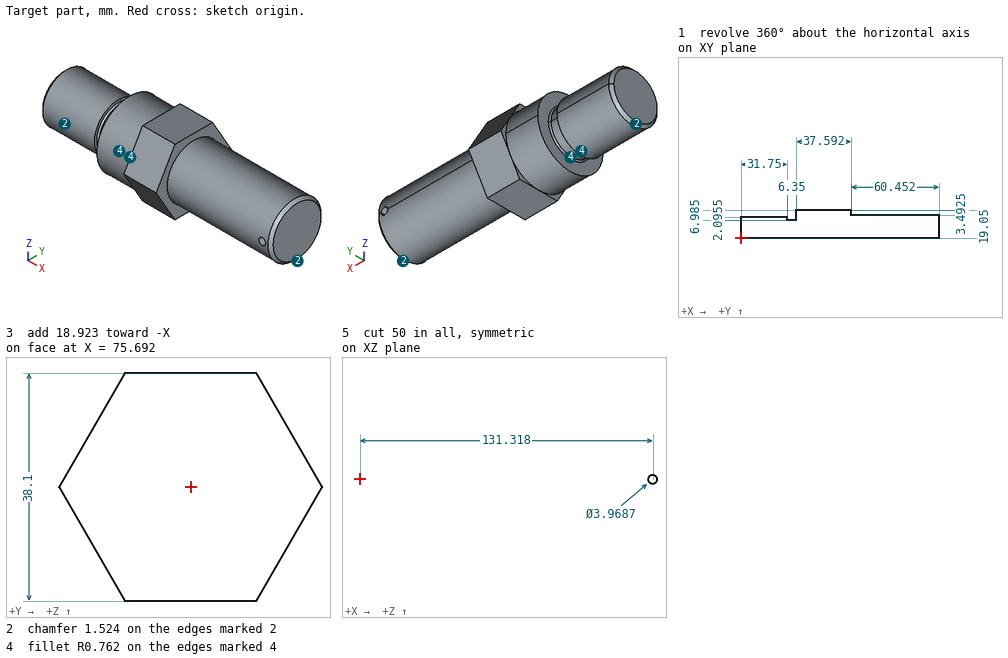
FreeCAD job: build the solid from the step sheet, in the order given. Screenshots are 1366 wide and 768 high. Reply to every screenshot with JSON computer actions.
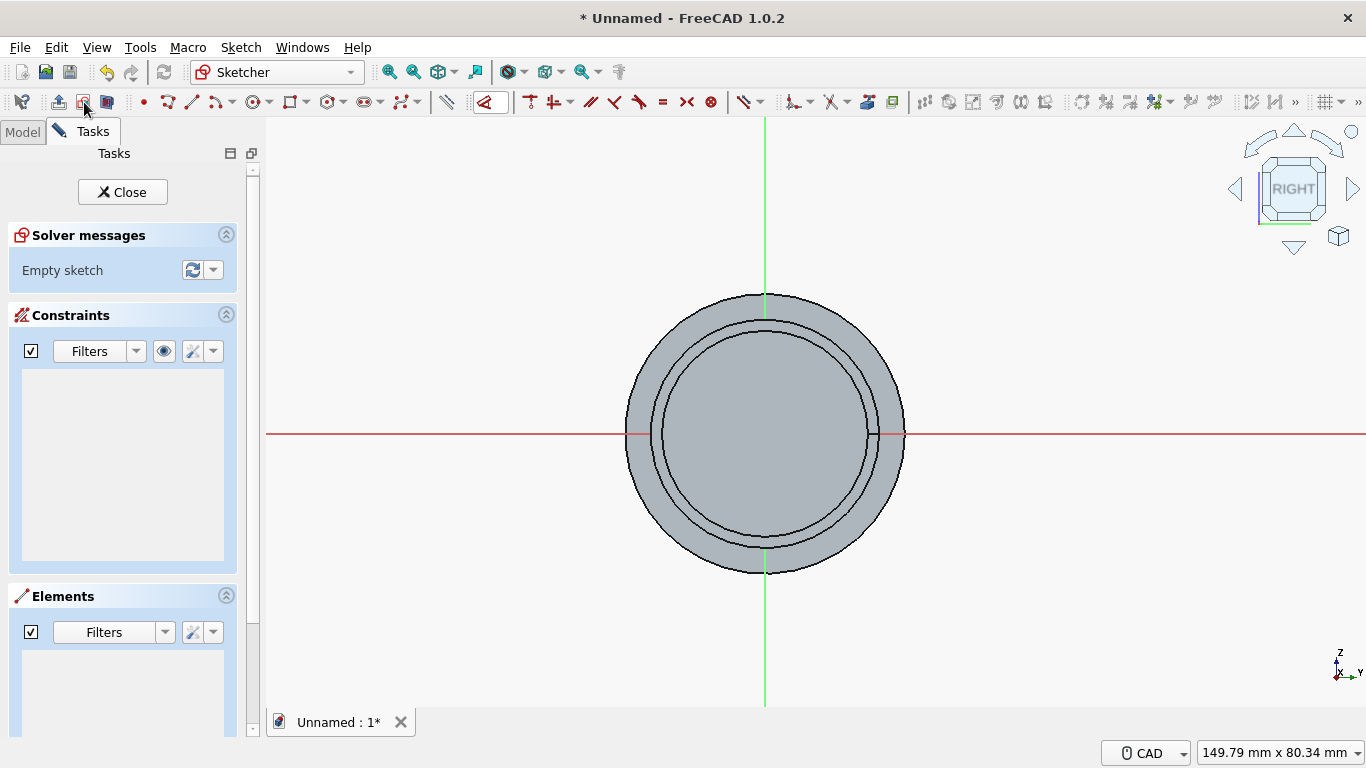
{"action": "key", "text": "q s"}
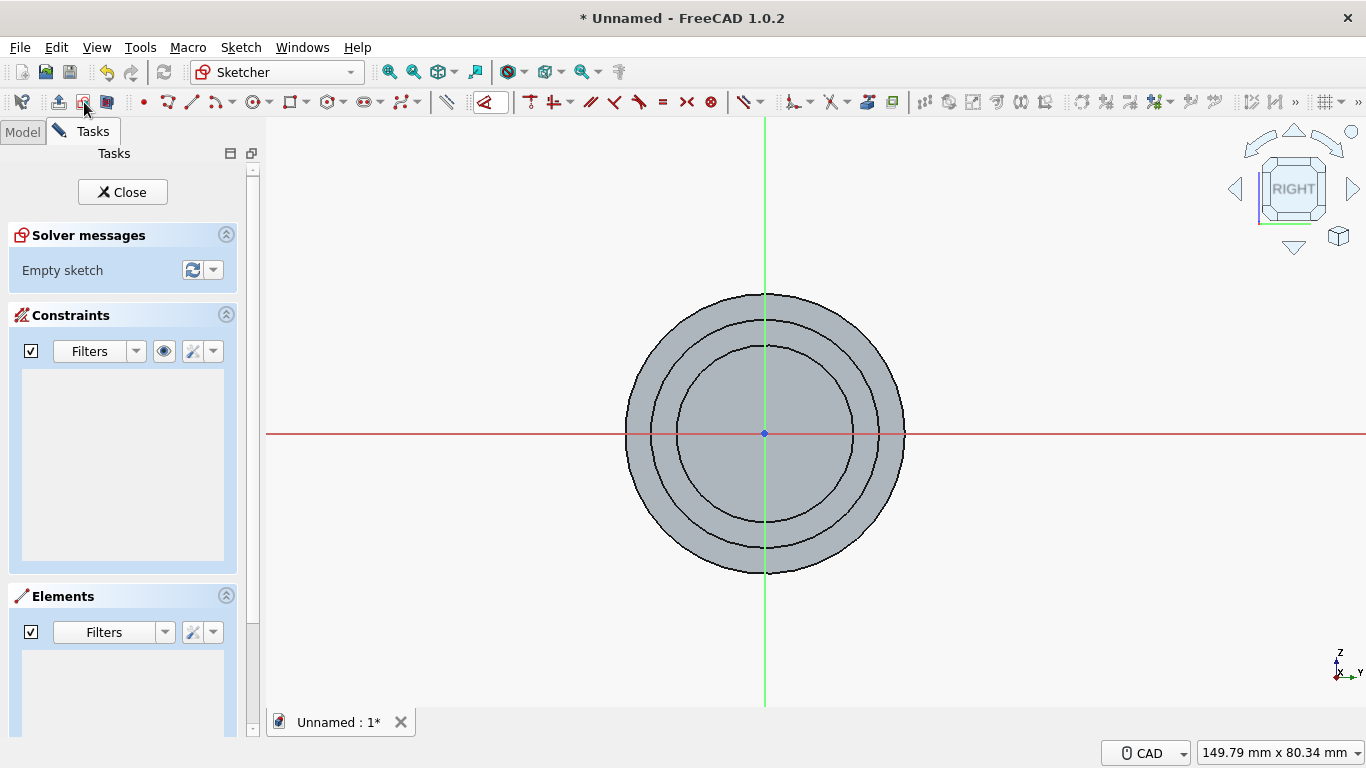
{"action": "key", "text": "g p 6"}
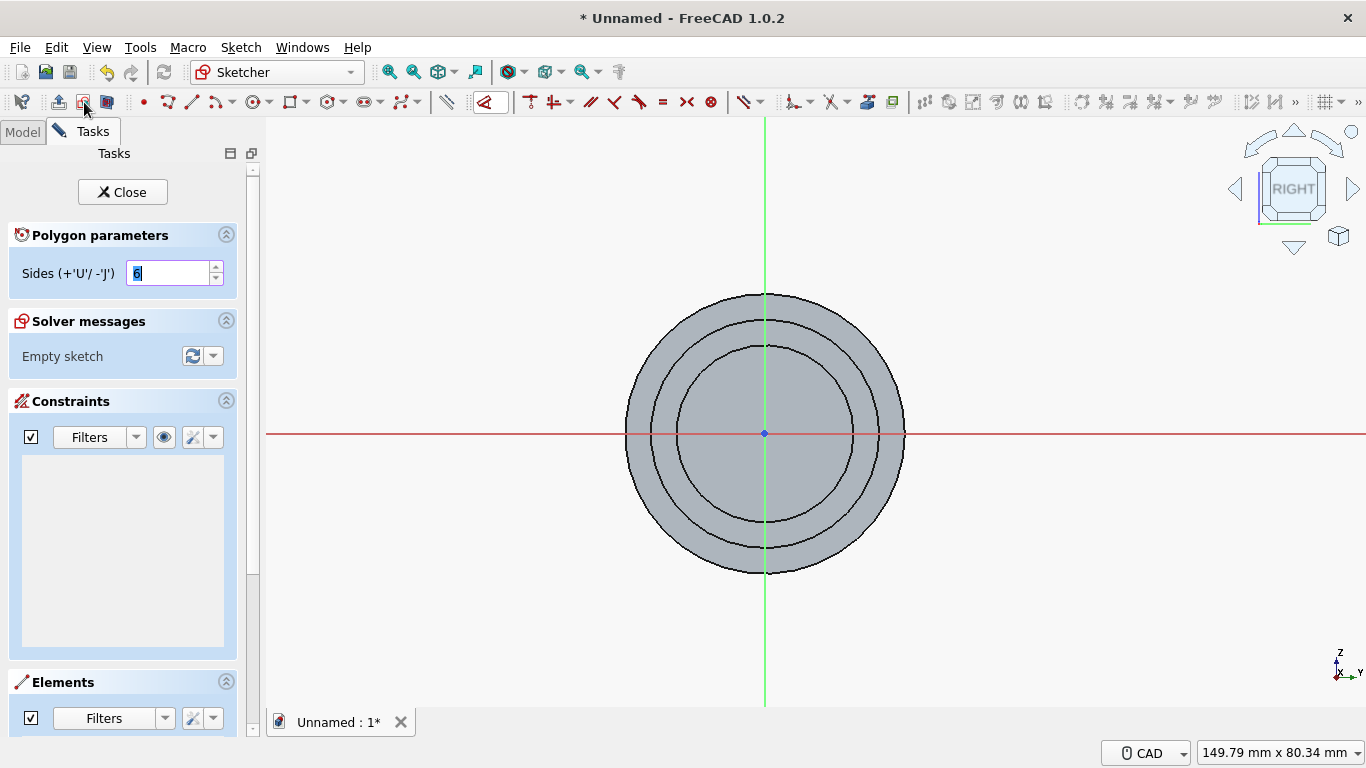
{"action": "left_click", "coordinate": [765, 434]}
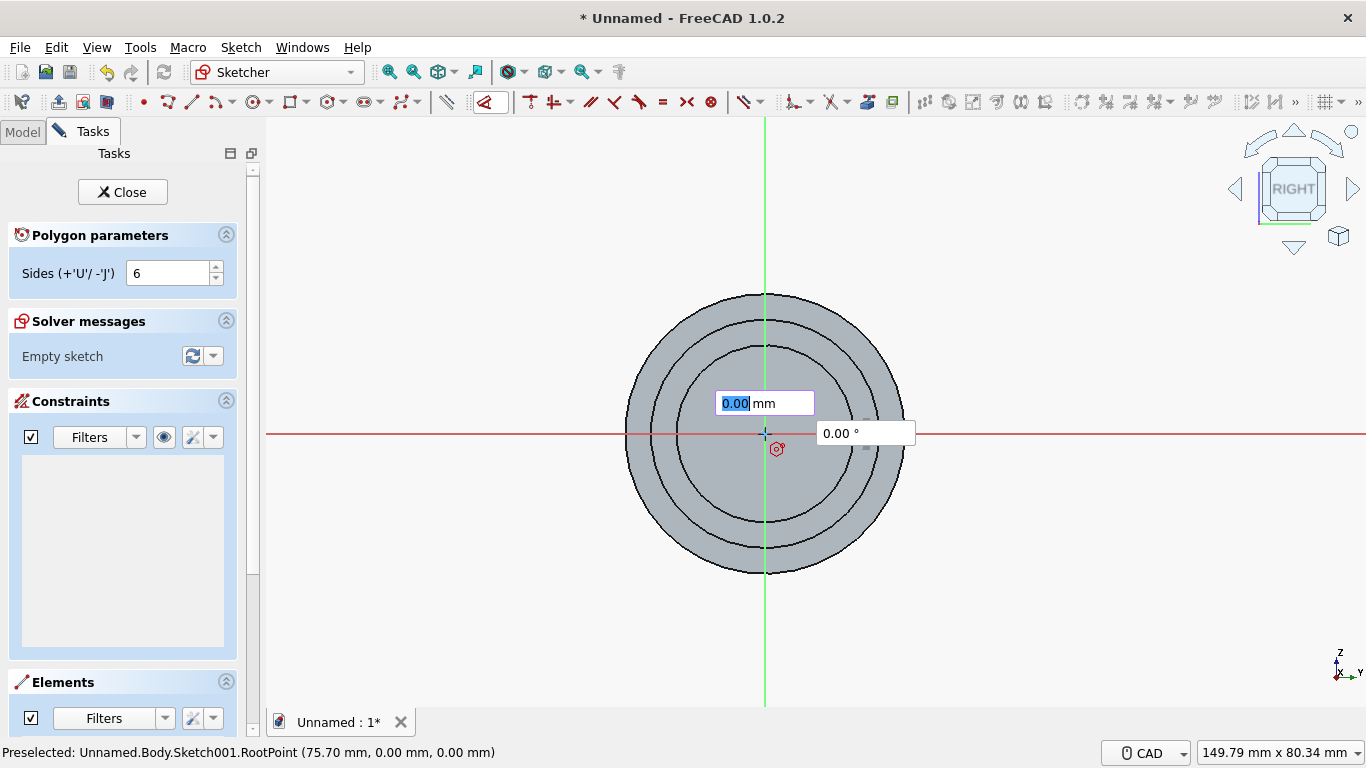
{"action": "left_click", "coordinate": [927, 434]}
{"action": "right_click", "coordinate": [927, 434]}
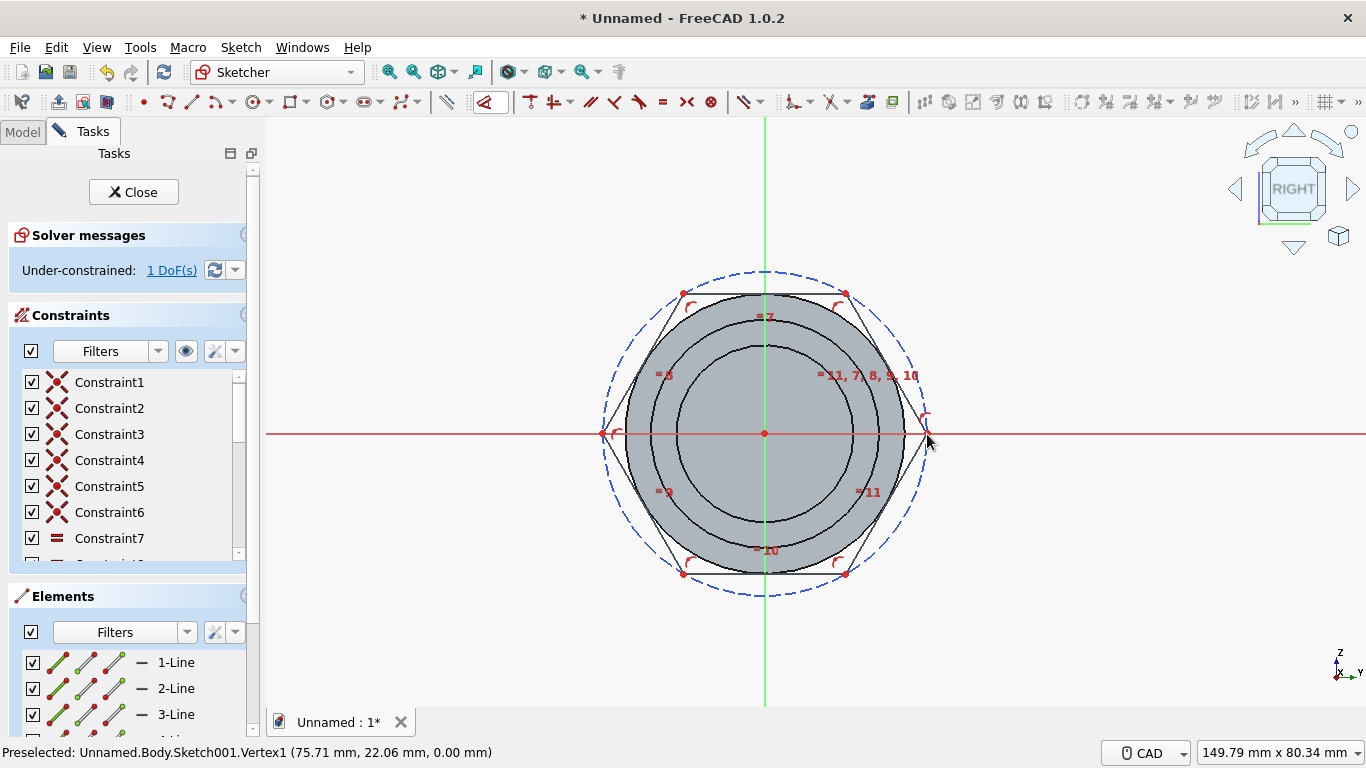
{"action": "left_click", "coordinate": [484, 102]}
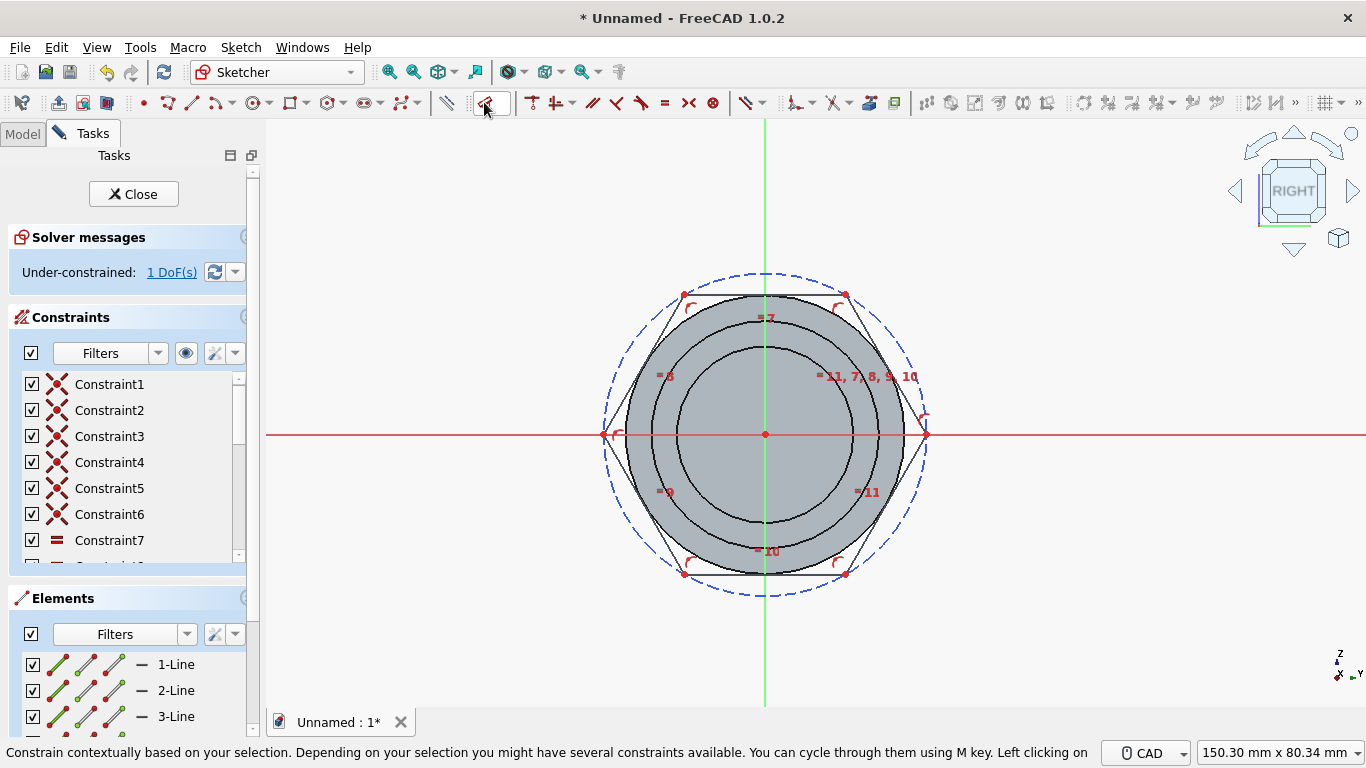
{"action": "left_click", "coordinate": [684, 575]}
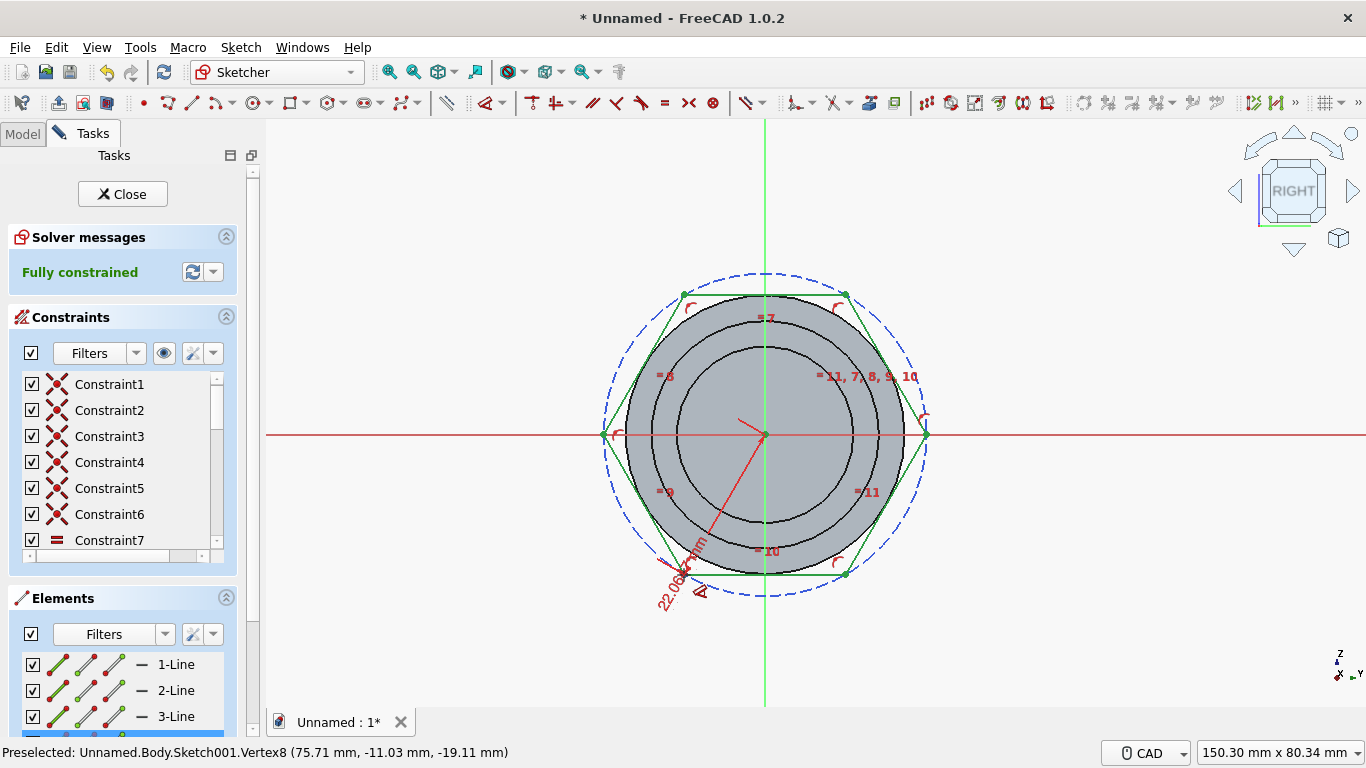
{"action": "left_click", "coordinate": [846, 295]}
{"action": "left_click", "coordinate": [928, 370]}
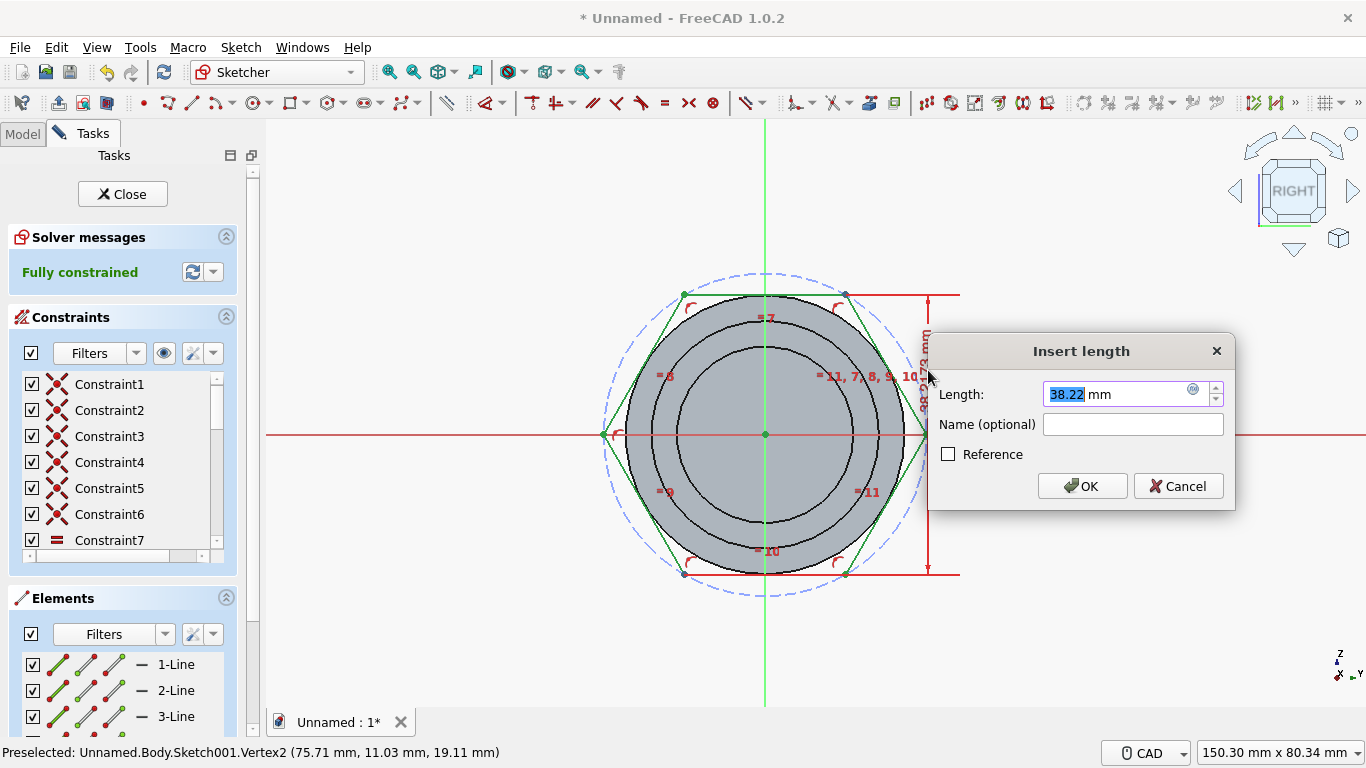
{"action": "type", "text": "38.1"}
{"action": "key", "text": "Return"}
{"action": "key", "text": "Escape"}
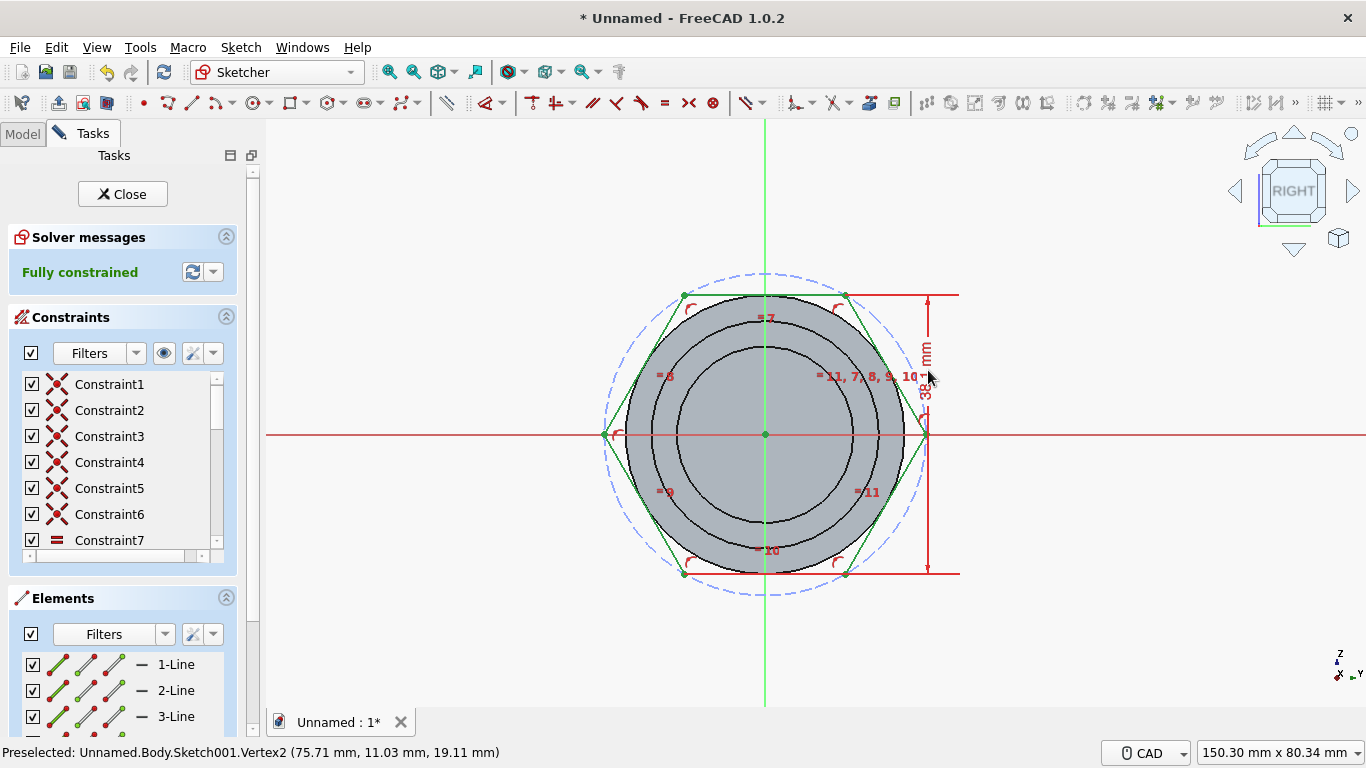
{"action": "left_click", "coordinate": [123, 194]}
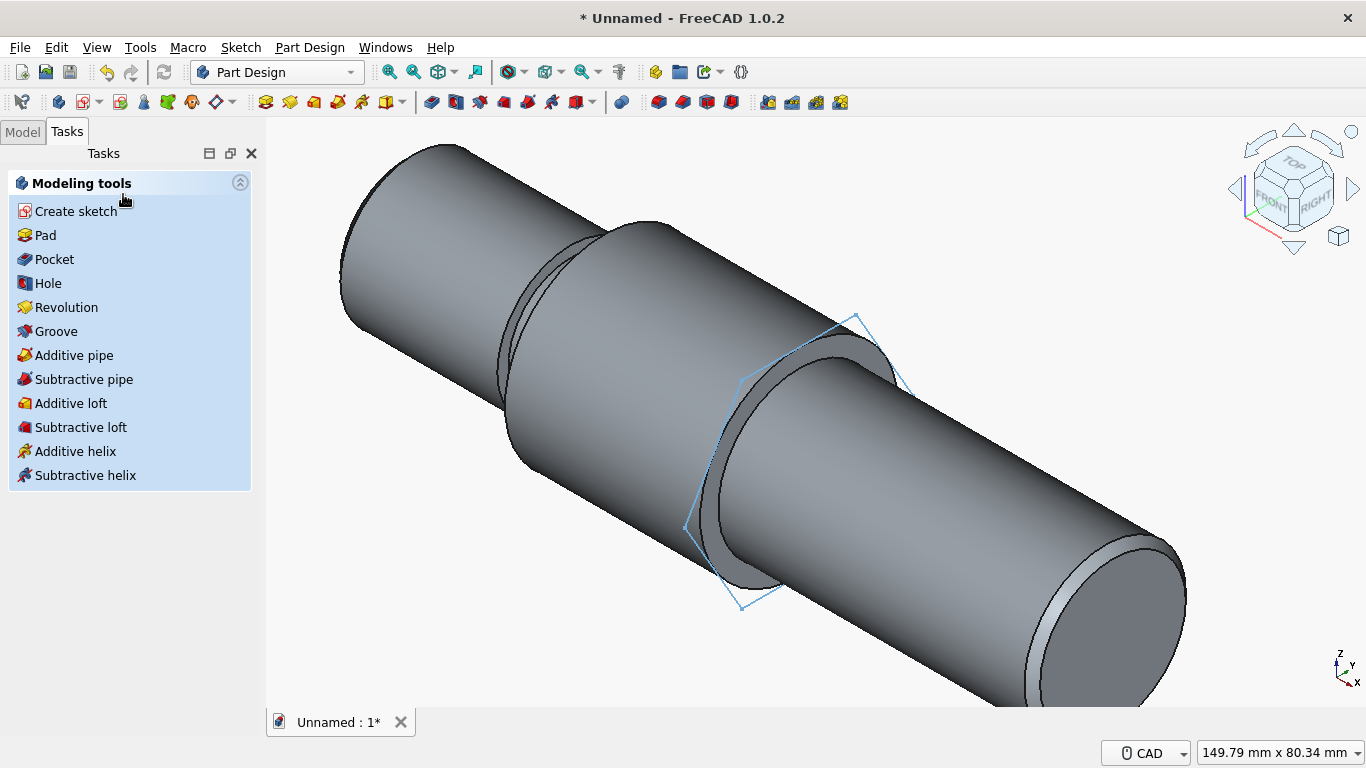
{"action": "left_click", "coordinate": [266, 102]}